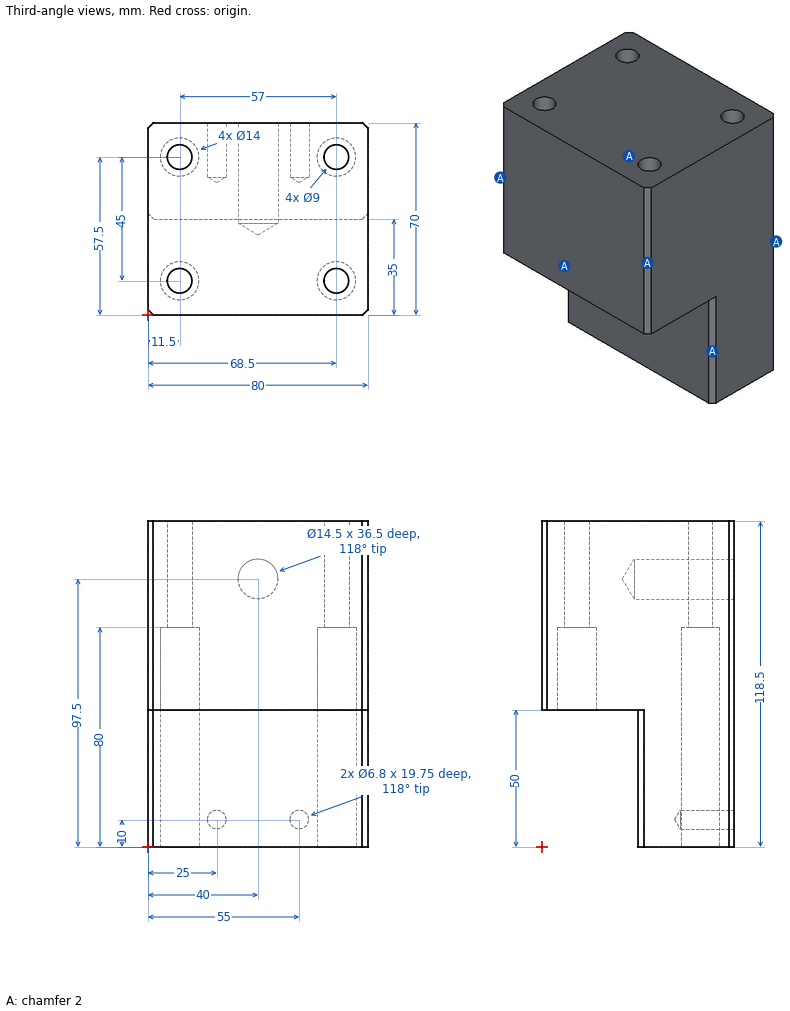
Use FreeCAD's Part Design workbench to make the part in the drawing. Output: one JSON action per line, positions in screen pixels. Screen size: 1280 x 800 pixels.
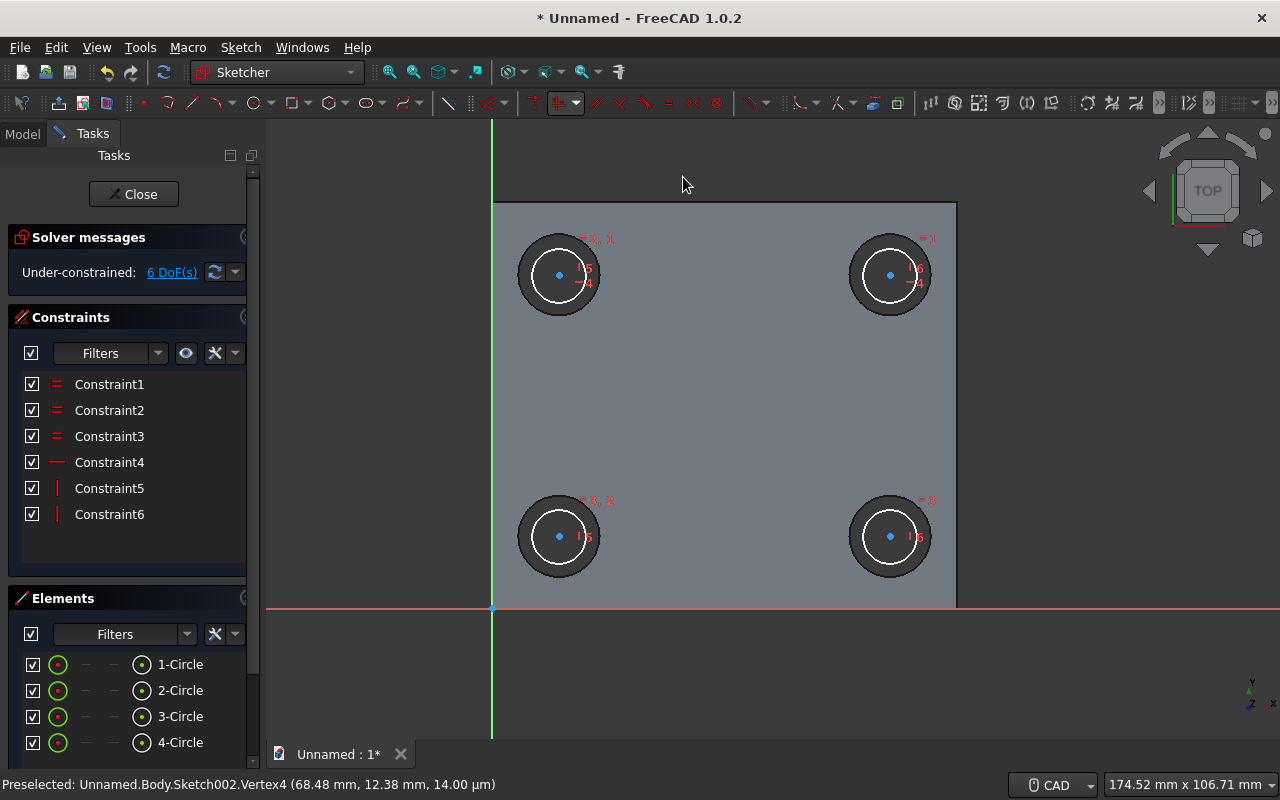
{"action": "left_click", "coordinate": [559, 537]}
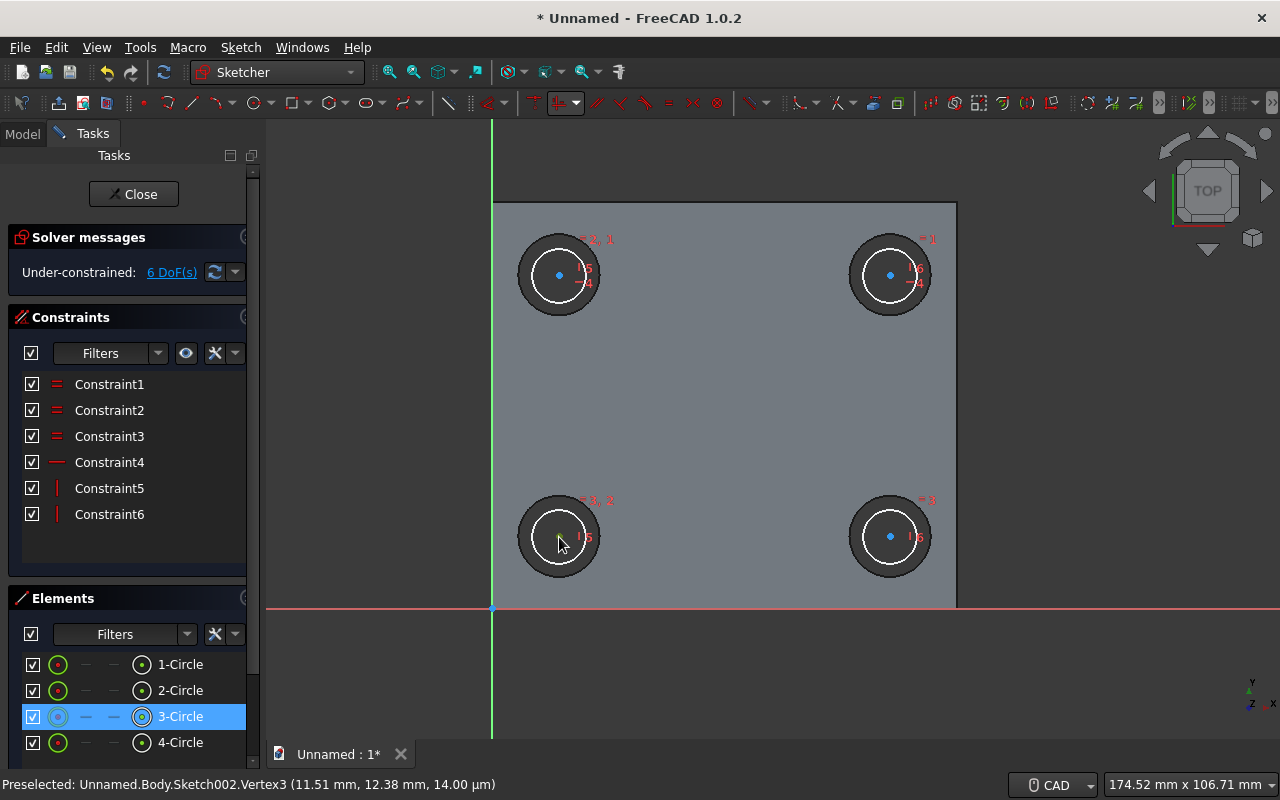
{"action": "left_click", "coordinate": [890, 537]}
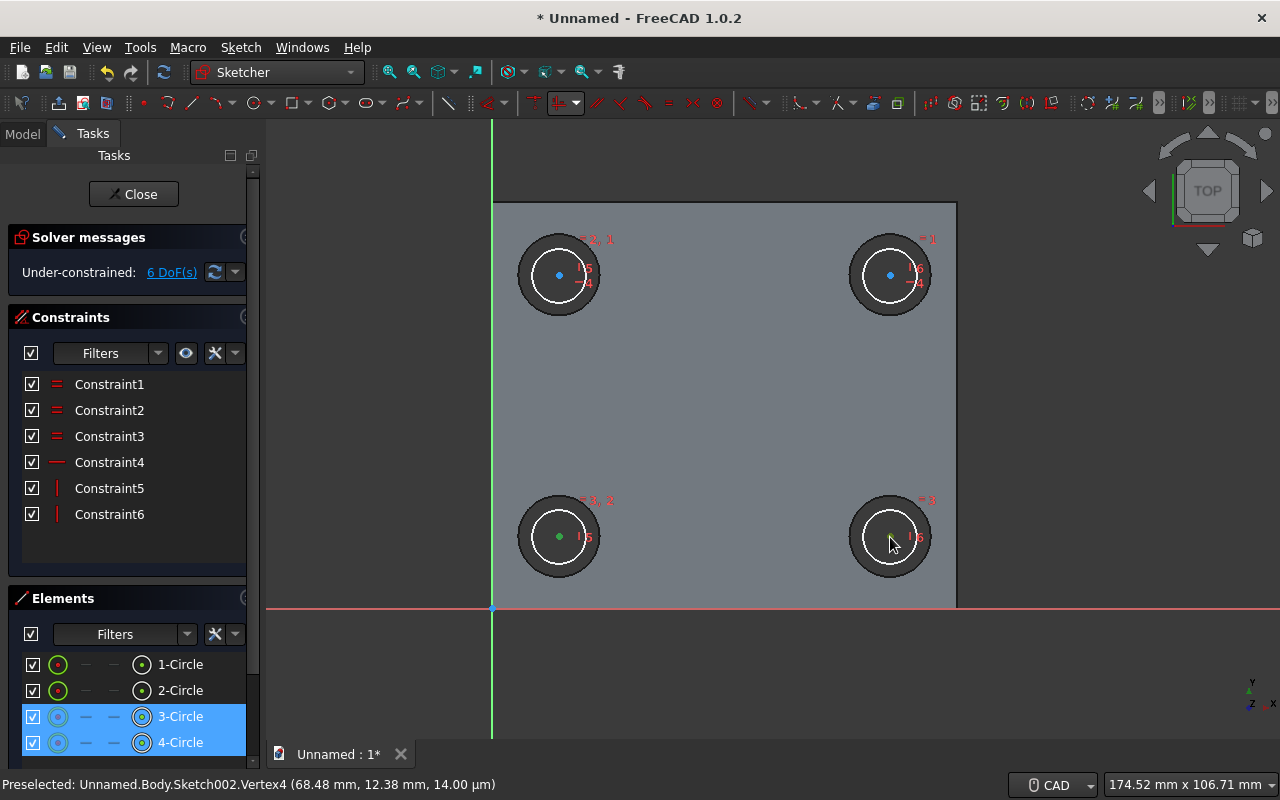
{"action": "left_click", "coordinate": [578, 104]}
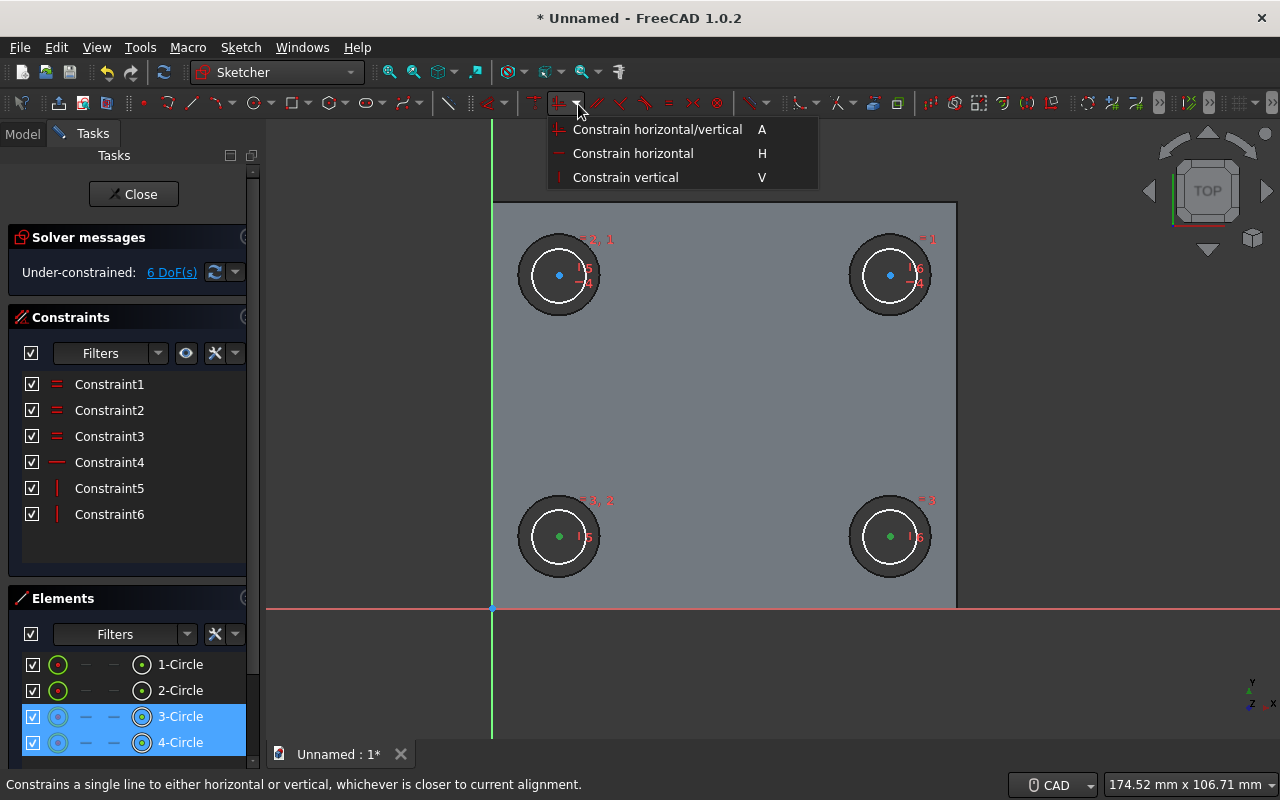
{"action": "left_click", "coordinate": [683, 153]}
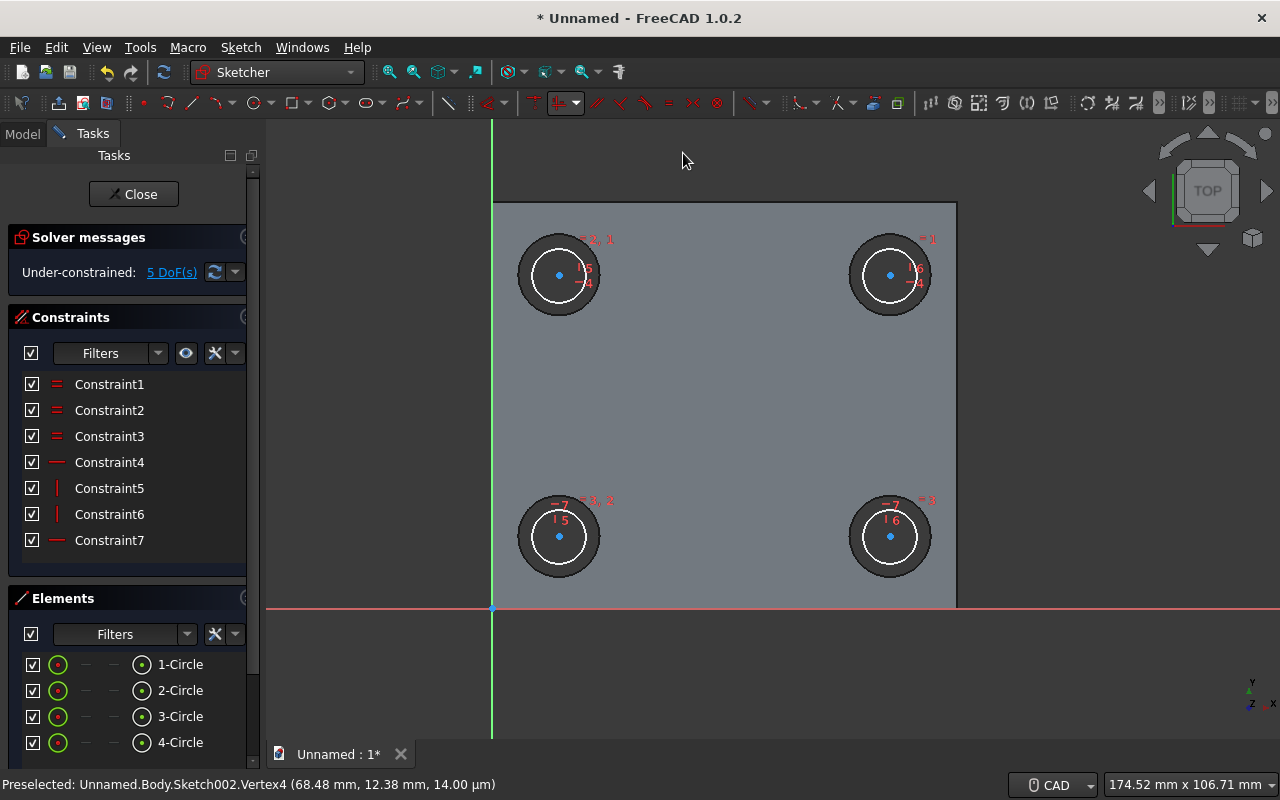
{"action": "key", "text": "d"}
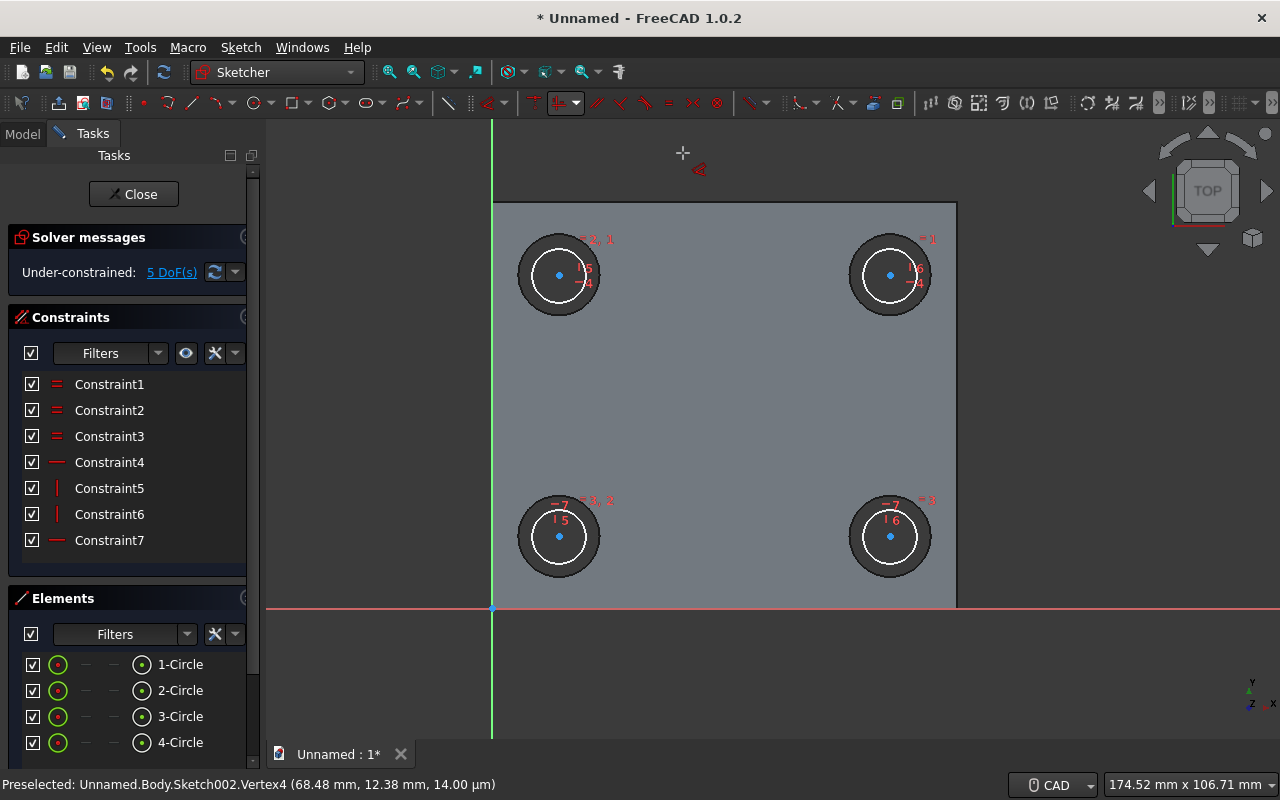
{"action": "left_click", "coordinate": [909, 257]}
{"action": "left_click", "coordinate": [932, 234]}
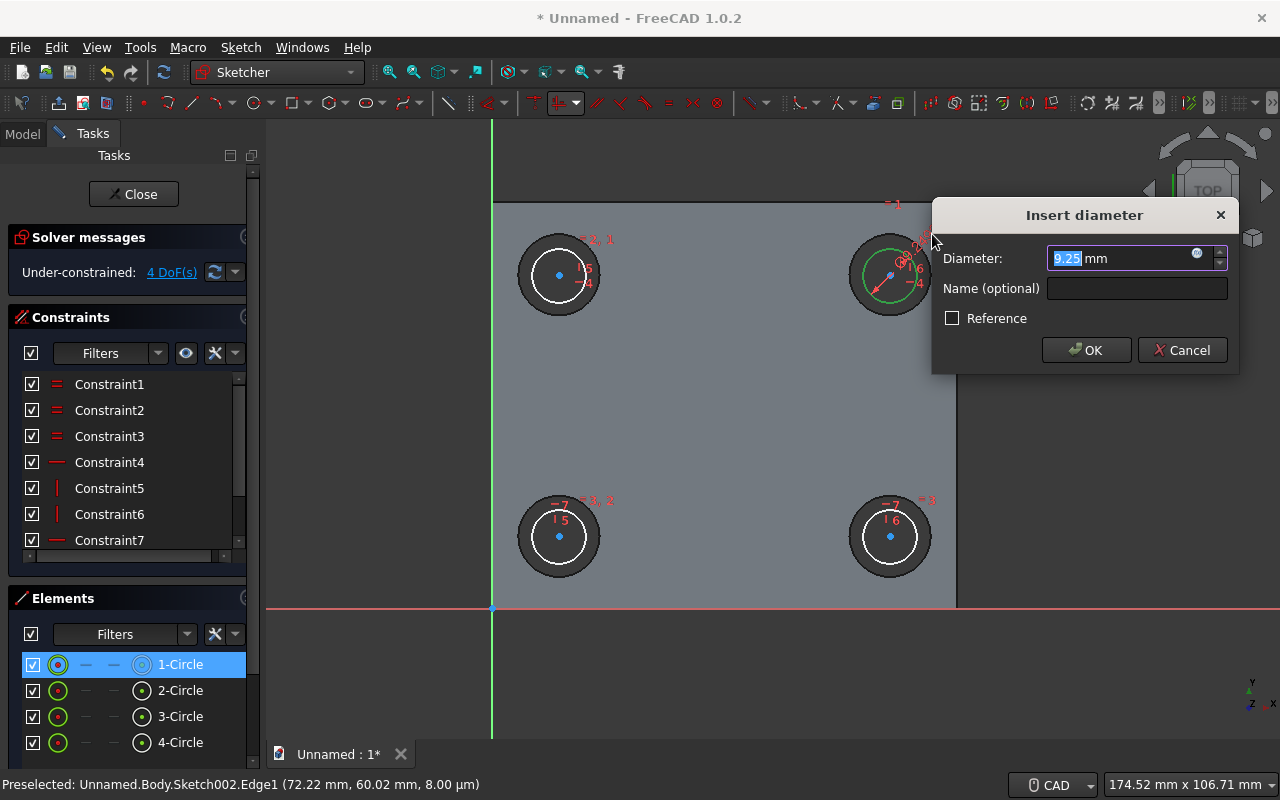
{"action": "type", "text": "9"}
{"action": "key", "text": "Return"}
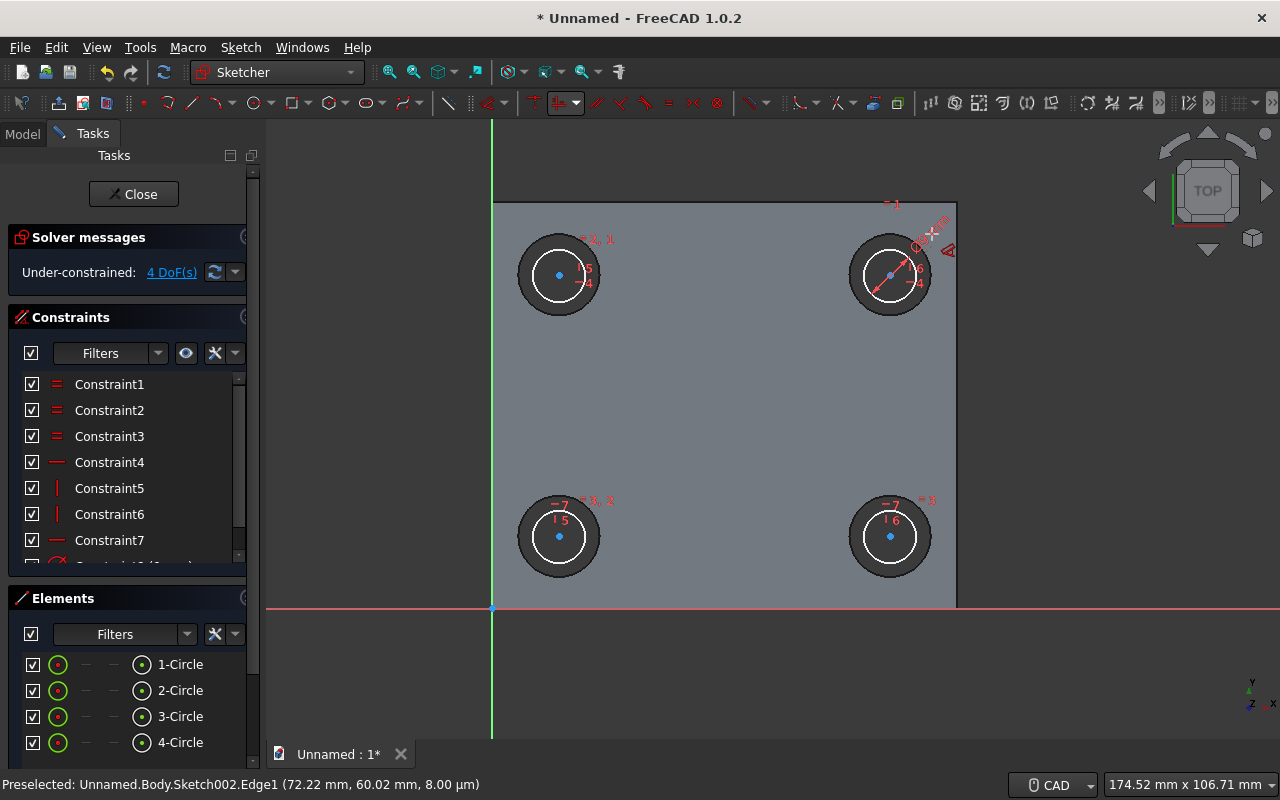
{"action": "left_click", "coordinate": [890, 276]}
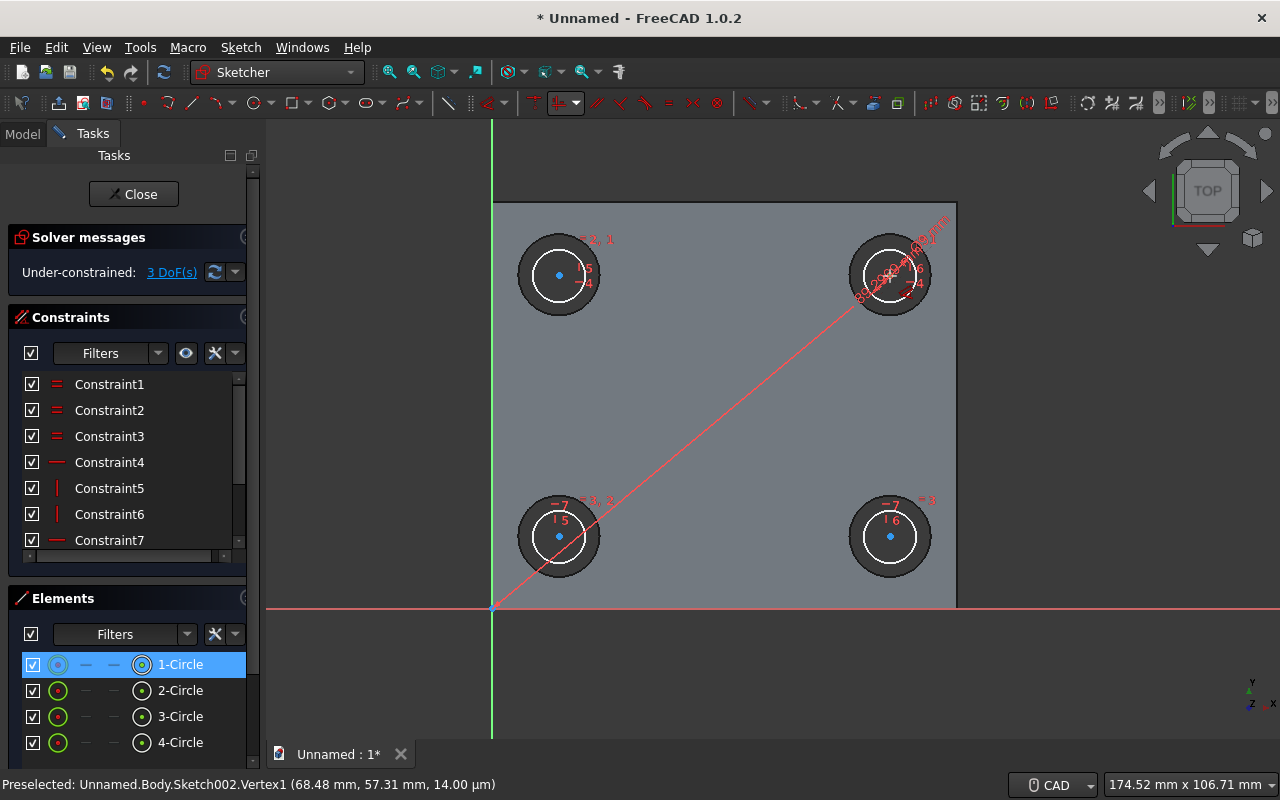
{"action": "left_click", "coordinate": [559, 276]}
{"action": "left_click", "coordinate": [725, 242]}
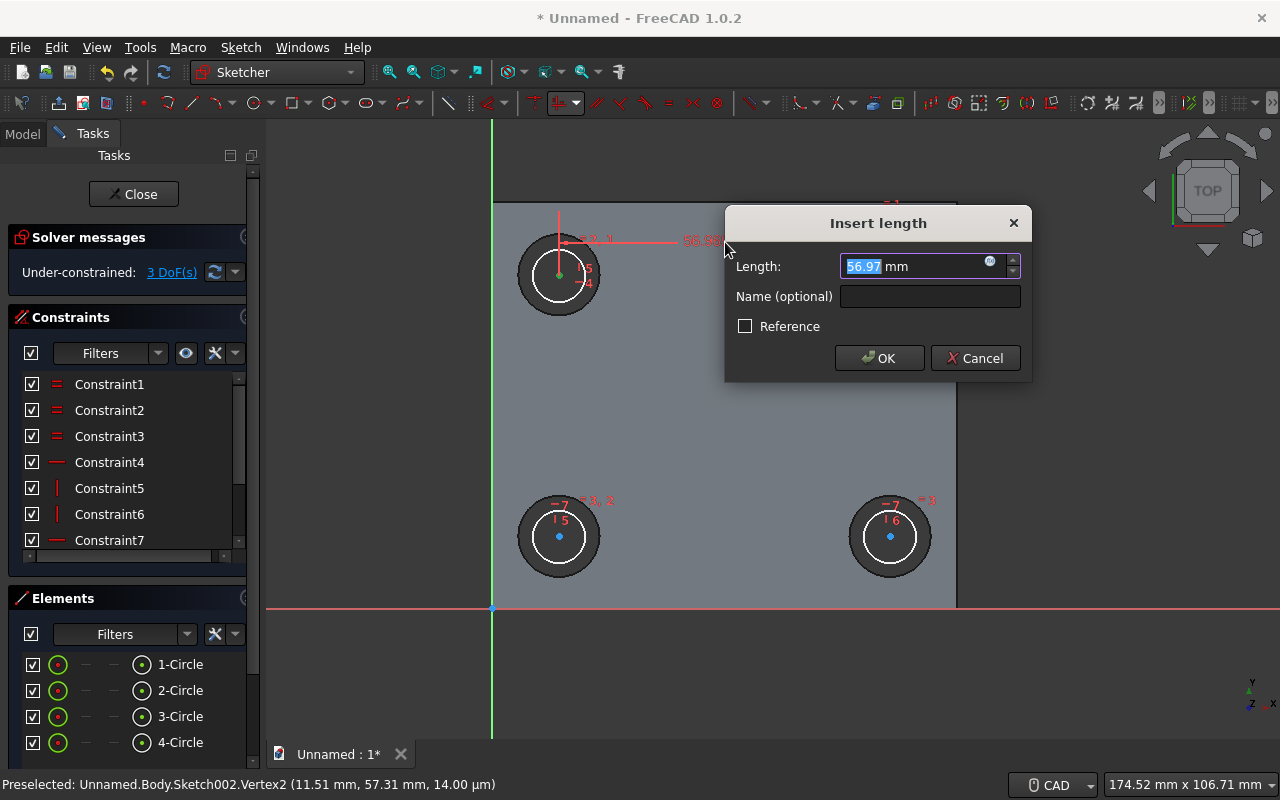
{"action": "type", "text": "57"}
{"action": "key", "text": "Return"}